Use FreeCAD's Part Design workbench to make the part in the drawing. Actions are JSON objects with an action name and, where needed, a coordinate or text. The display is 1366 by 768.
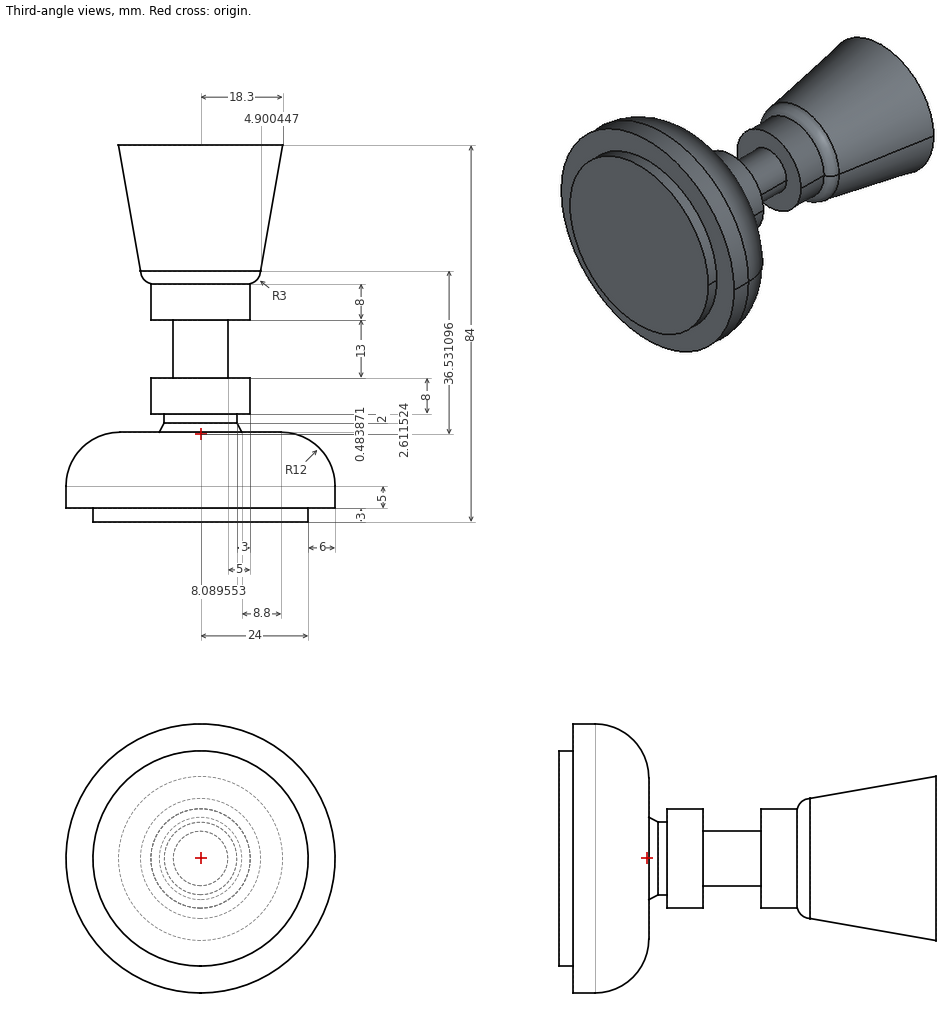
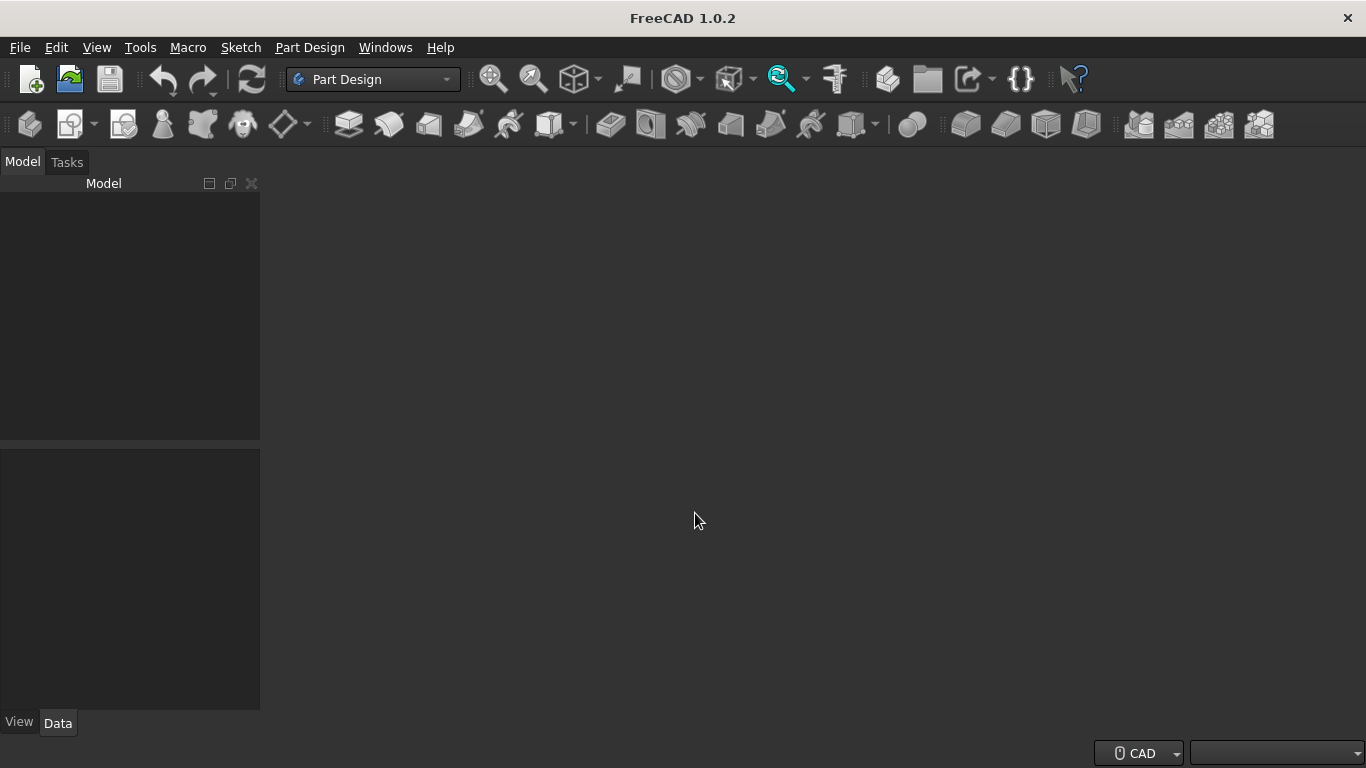
{"action": "key", "text": "ctrl+n"}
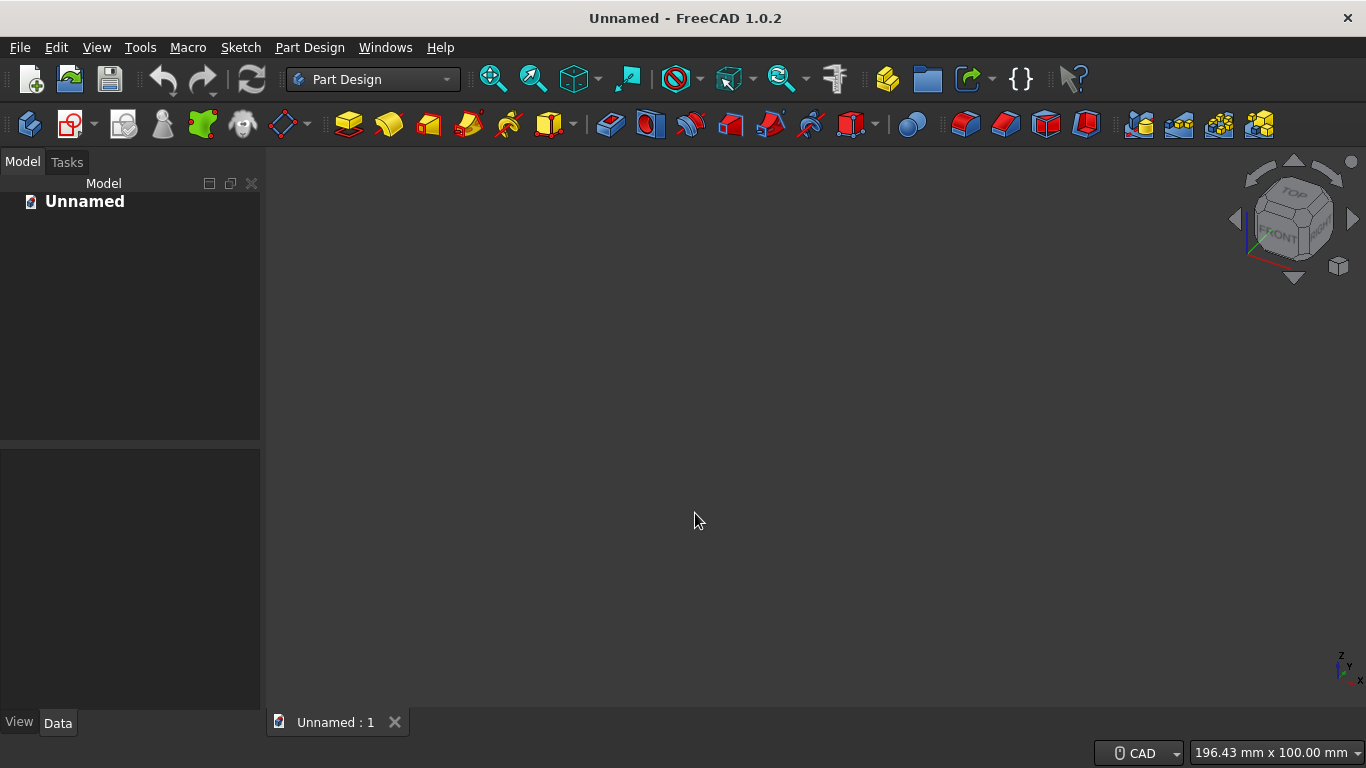
{"action": "left_click", "coordinate": [70, 124]}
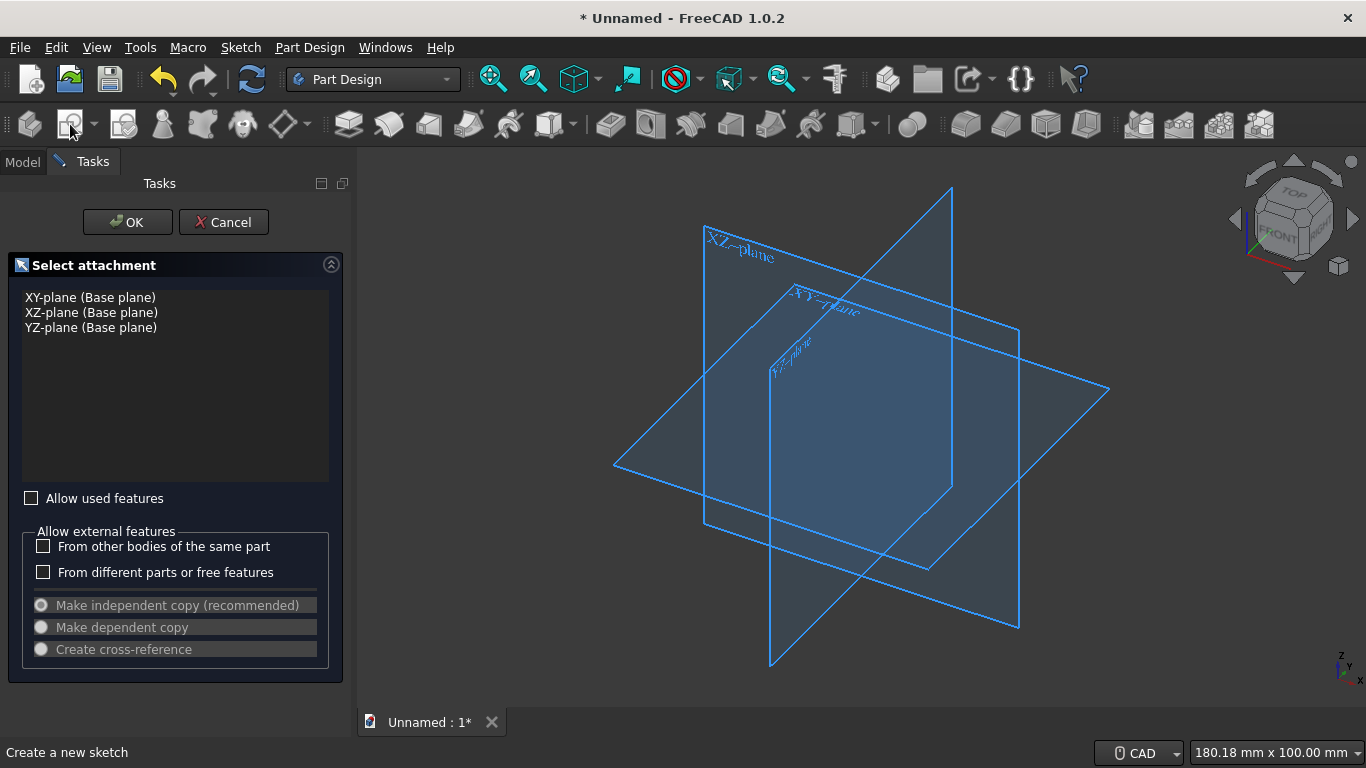
{"action": "left_click", "coordinate": [82, 298]}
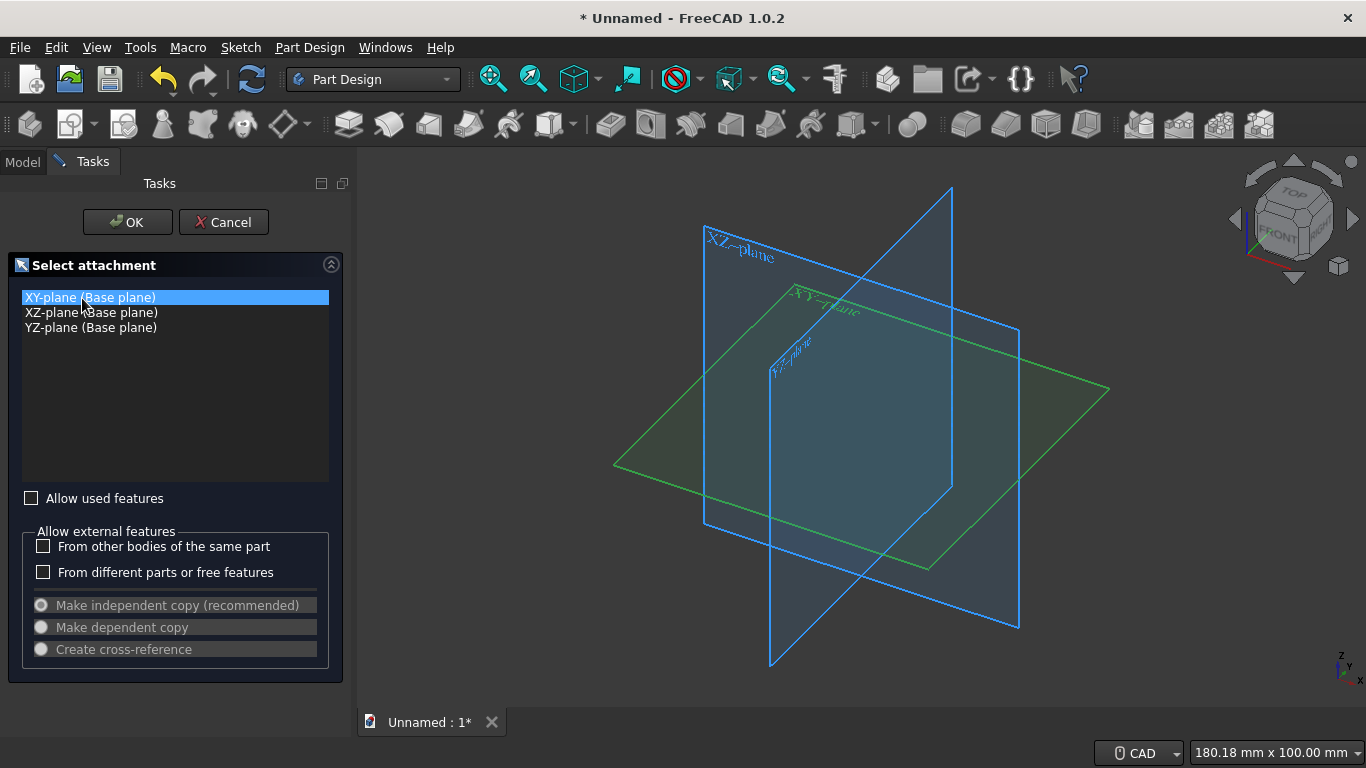
{"action": "left_click", "coordinate": [128, 222]}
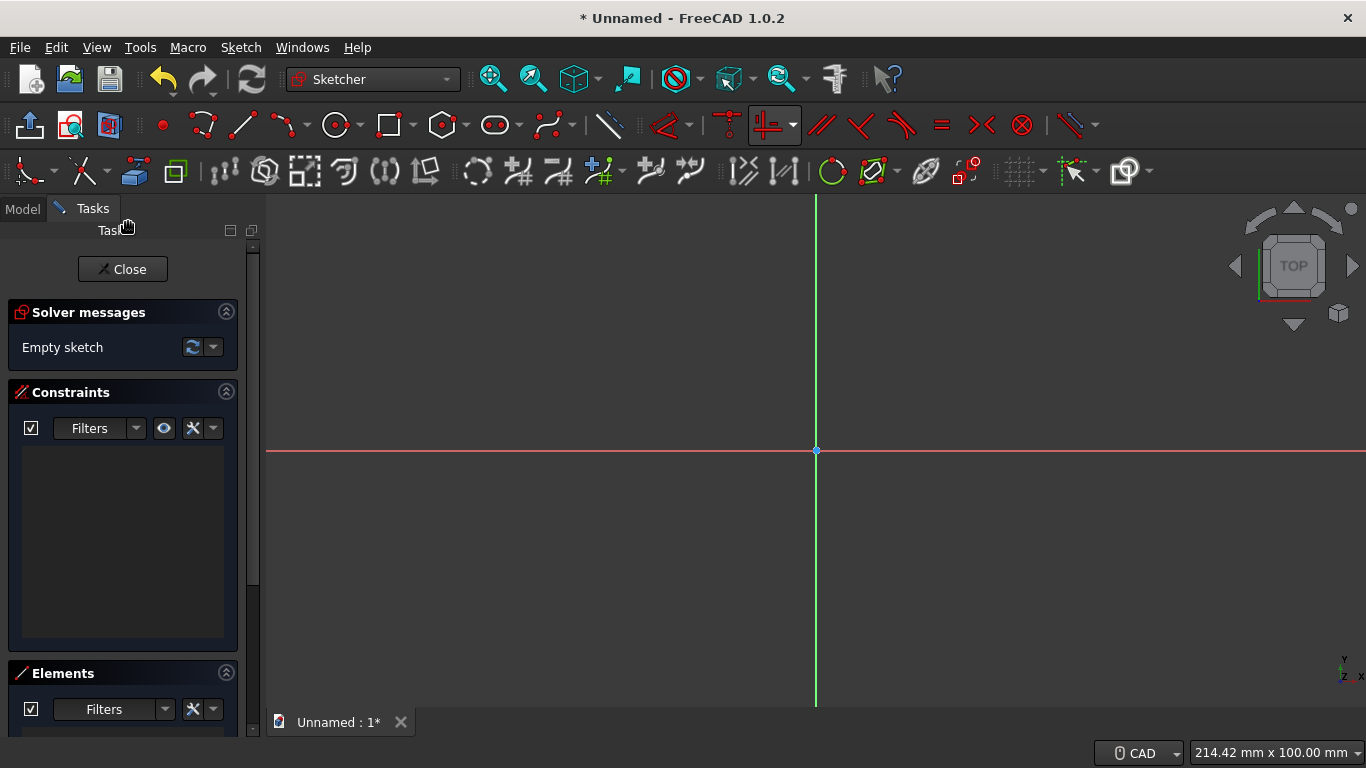
{"action": "scroll", "coordinate": [452, 679], "scroll_direction": "down", "scroll_amount": 2}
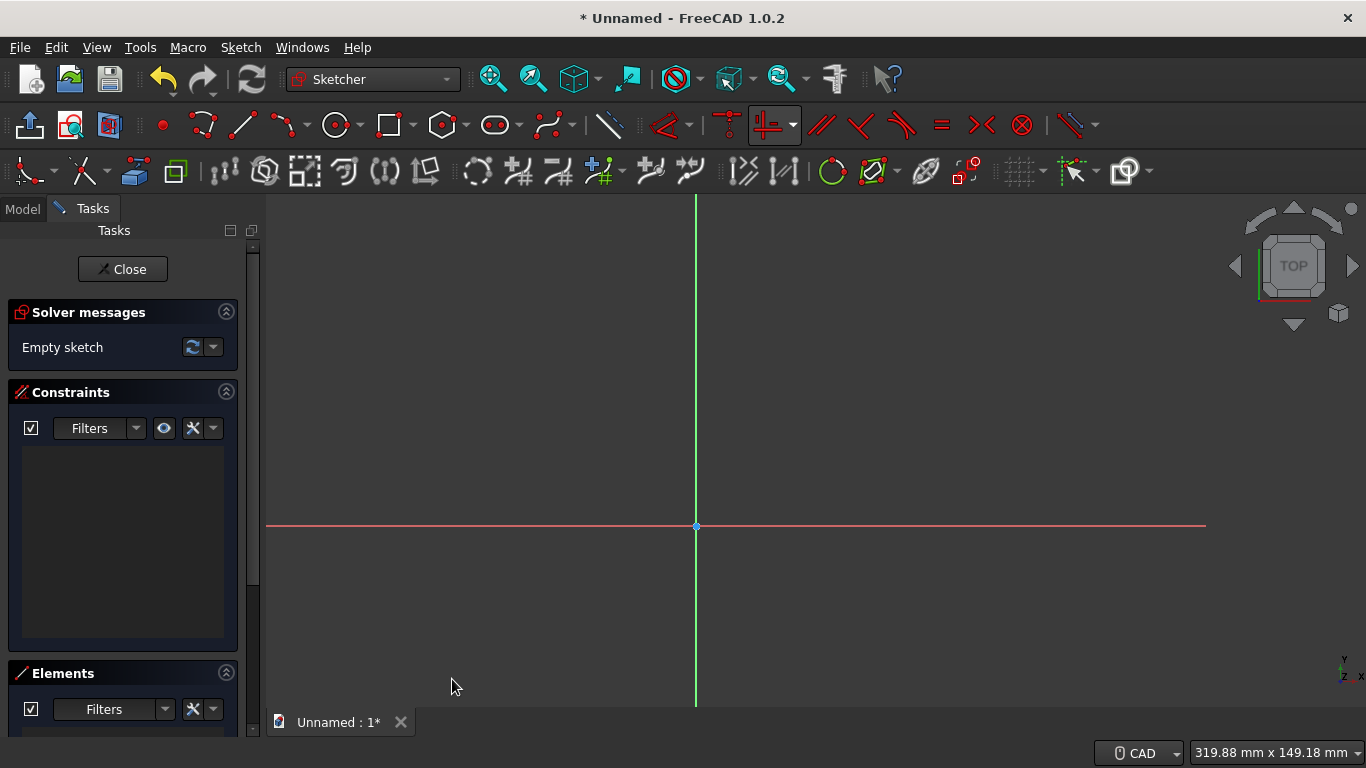
{"action": "key", "text": "g m"}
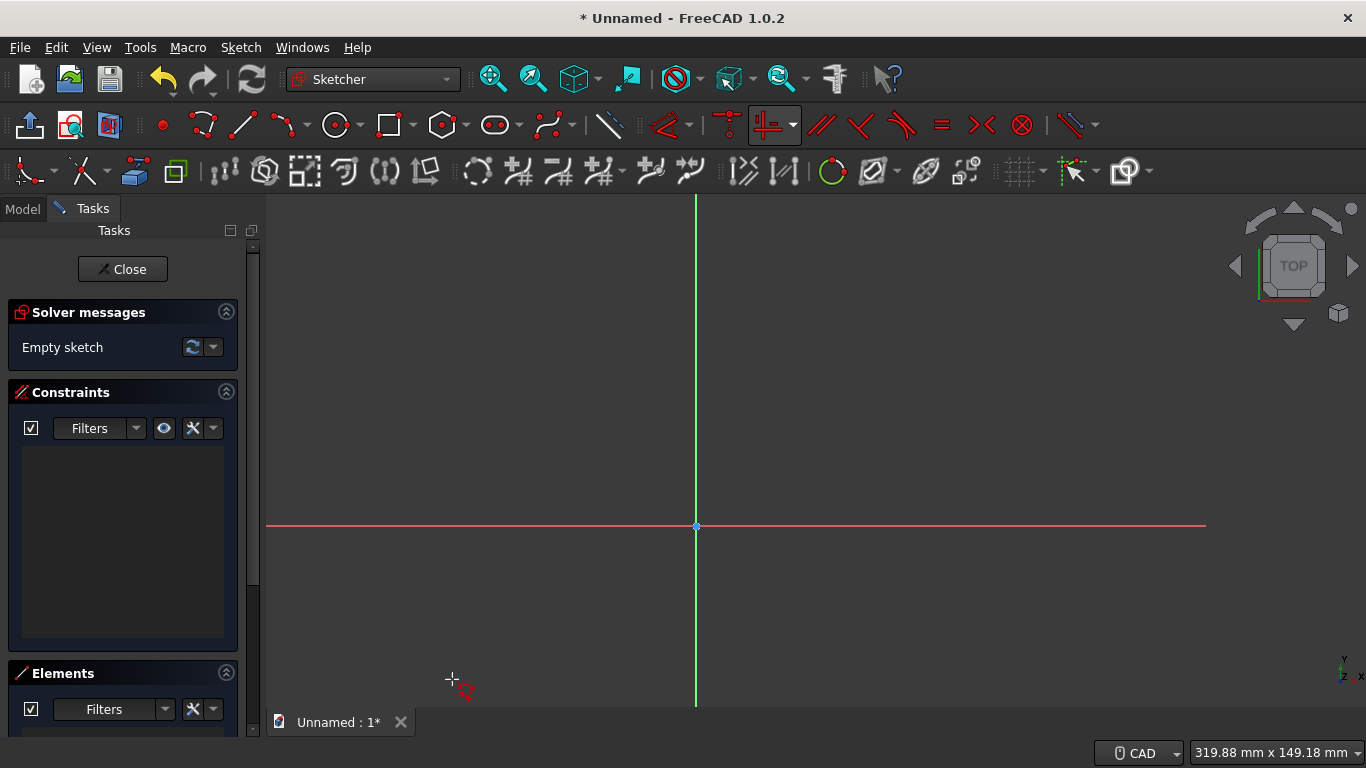
{"action": "scroll", "coordinate": [758, 524], "scroll_direction": "up", "scroll_amount": 12}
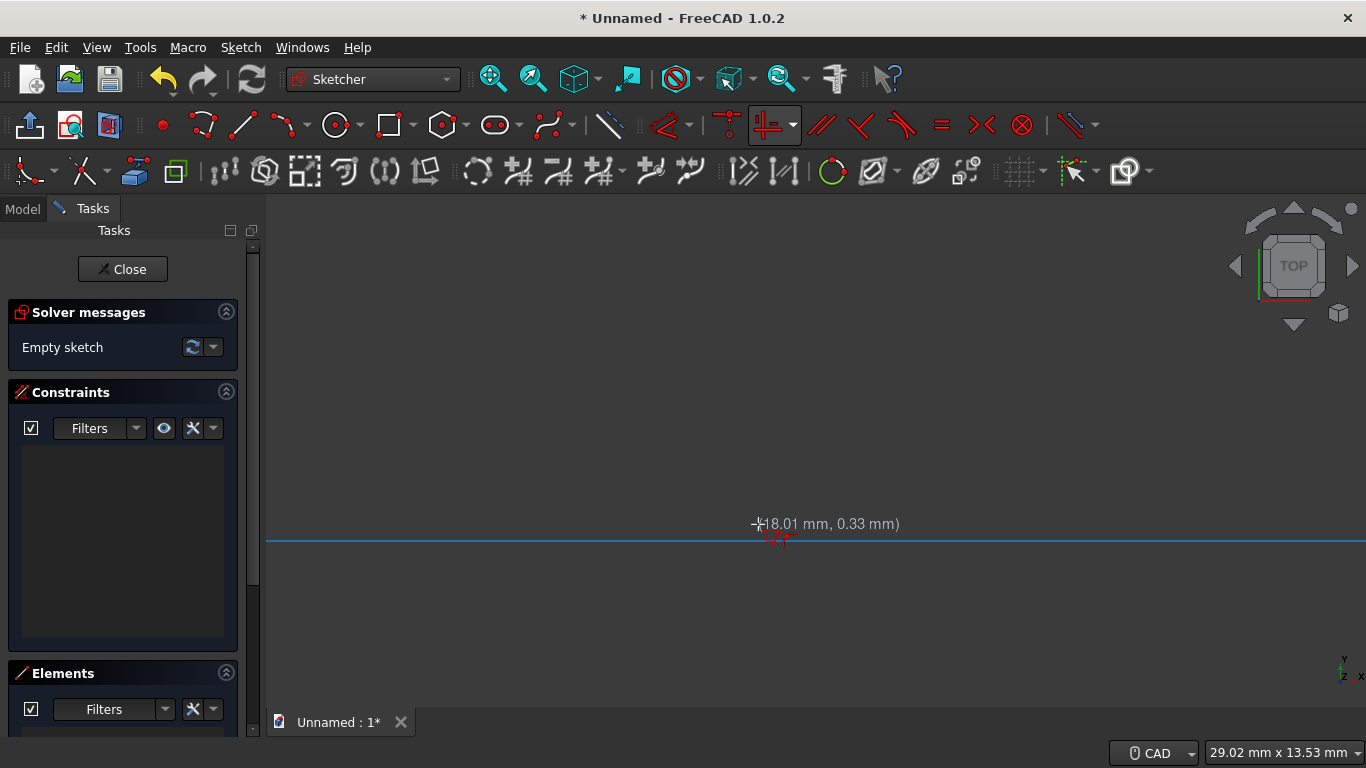
{"action": "left_click", "coordinate": [753, 523]}
{"action": "left_click", "coordinate": [419, 523]}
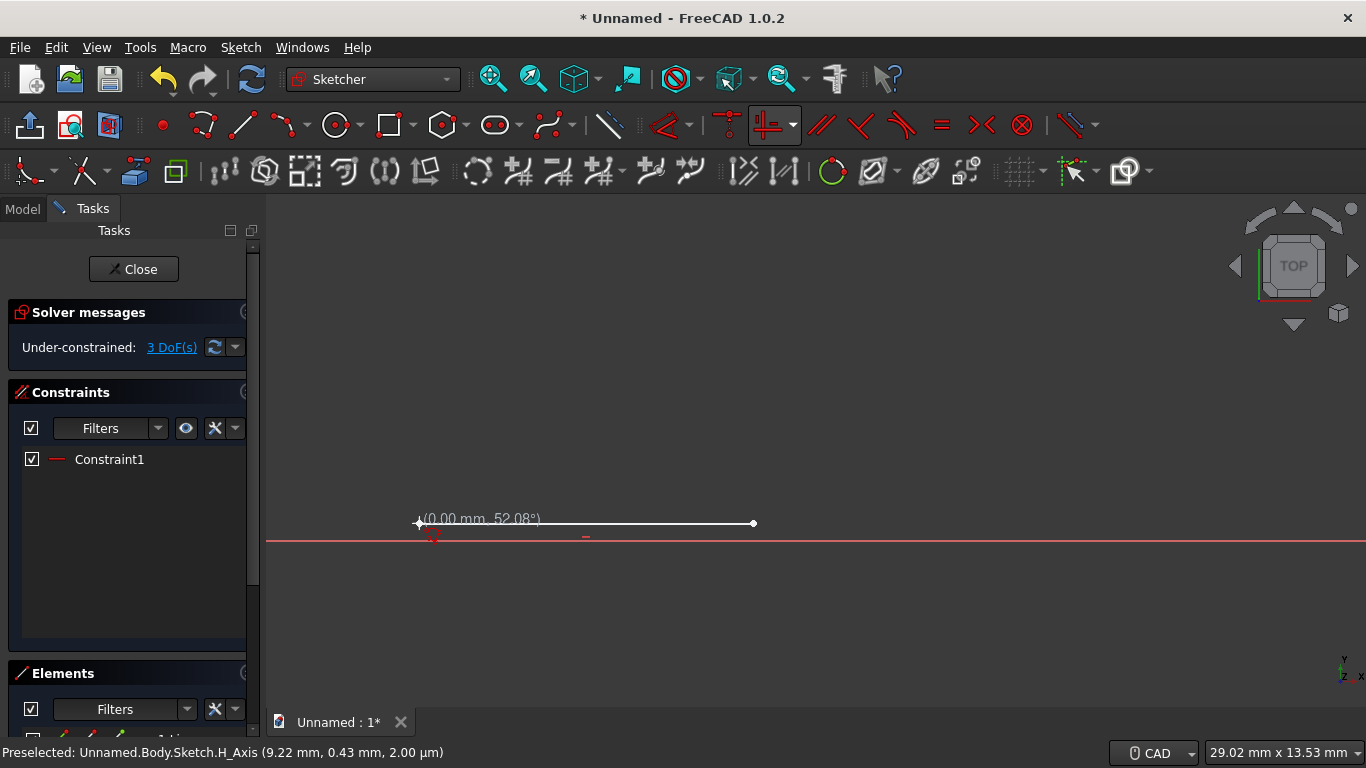
{"action": "scroll", "coordinate": [761, 545], "scroll_direction": "down", "scroll_amount": 11}